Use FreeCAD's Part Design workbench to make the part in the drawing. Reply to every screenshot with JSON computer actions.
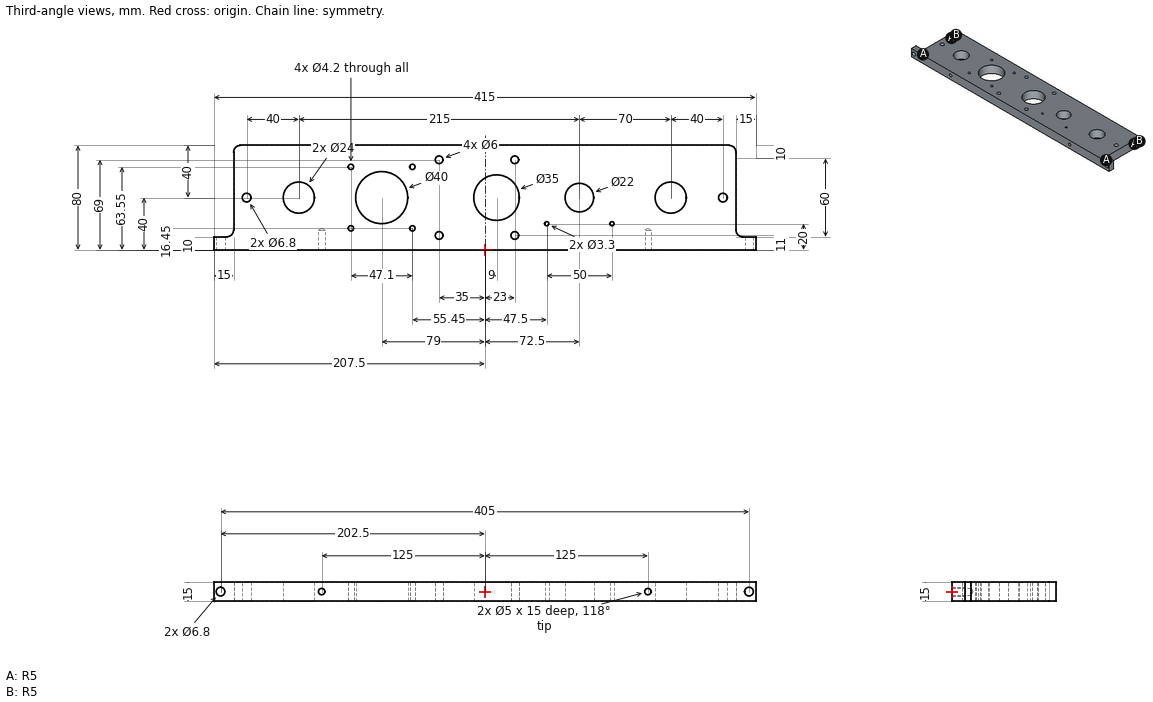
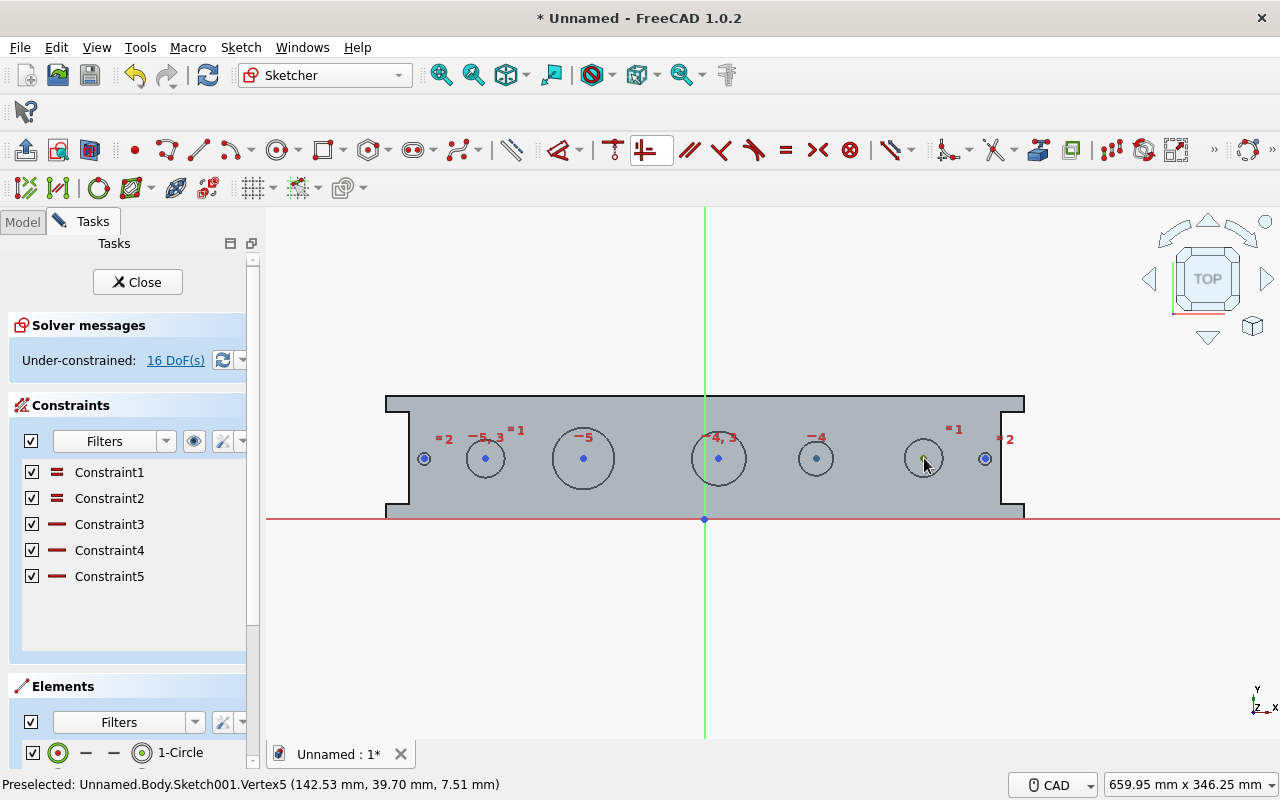
{"action": "left_click", "coordinate": [668, 150]}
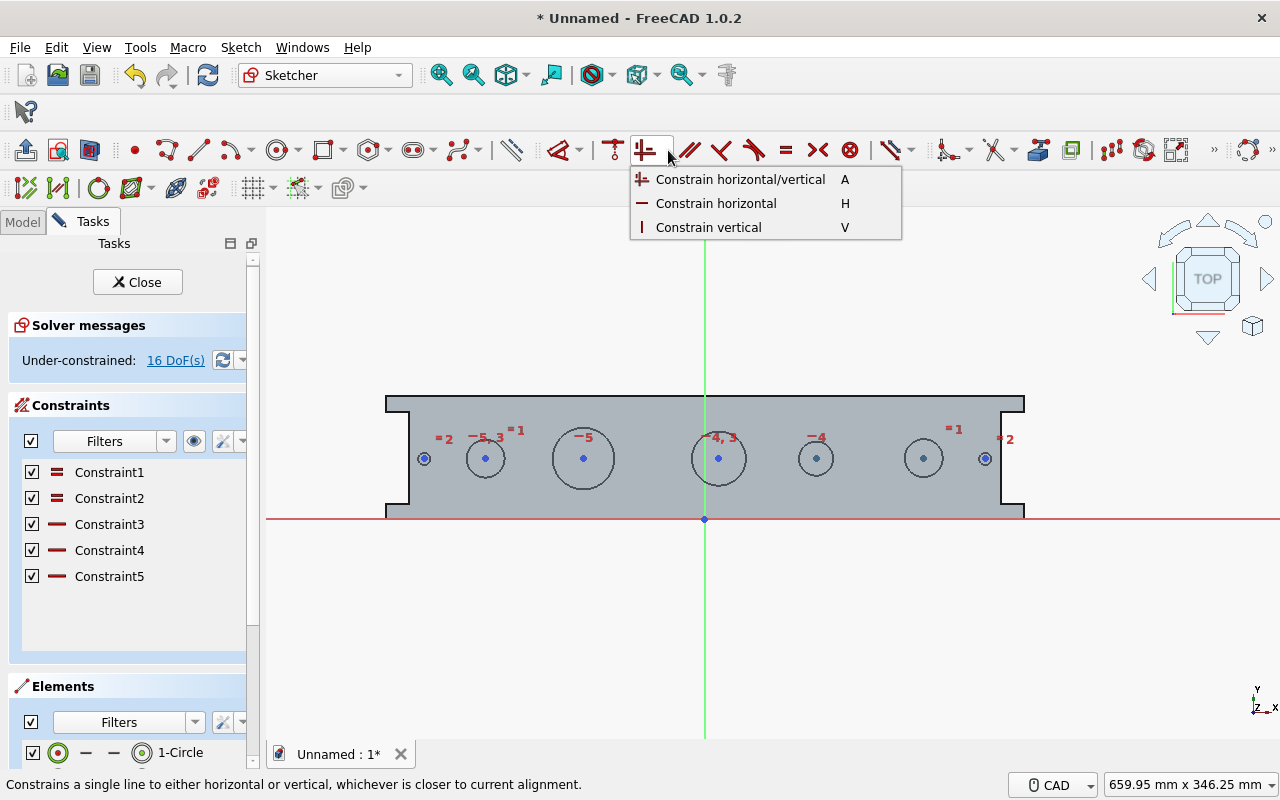
{"action": "left_click", "coordinate": [766, 203]}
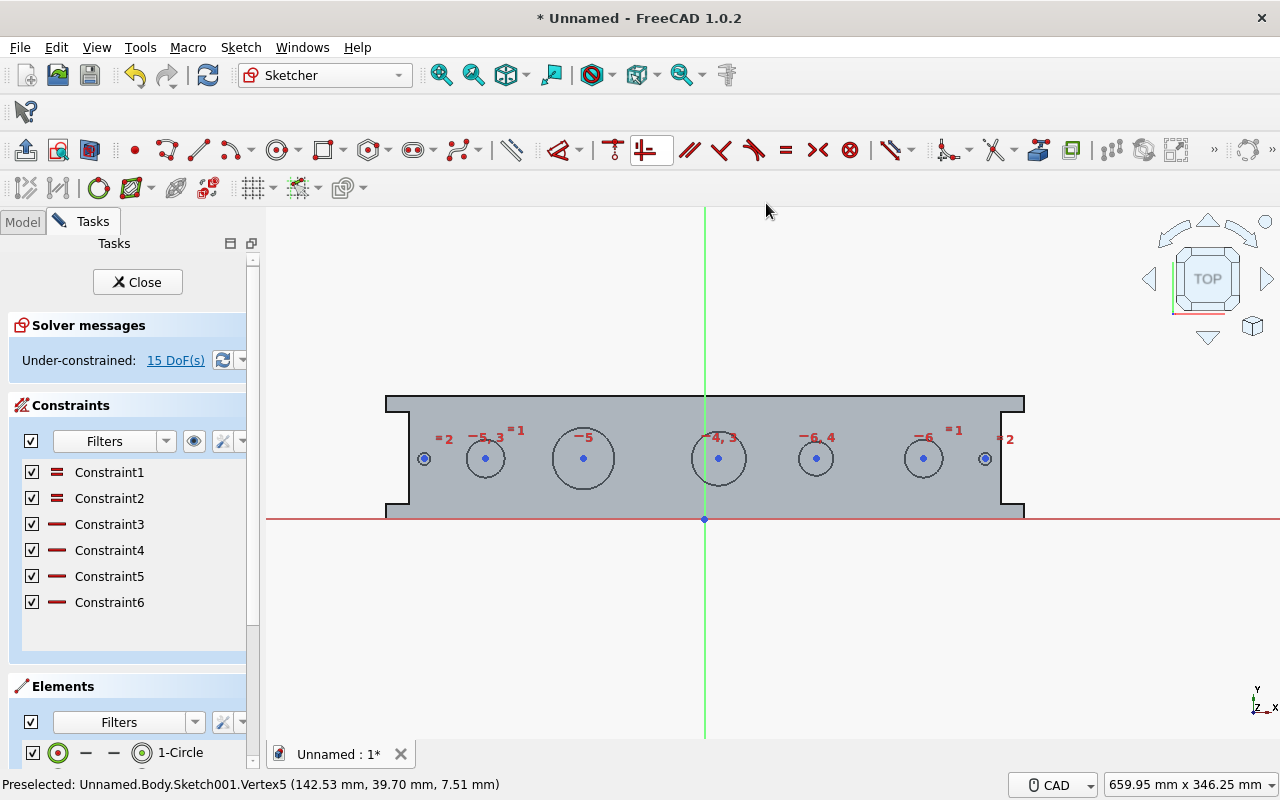
{"action": "left_click", "coordinate": [486, 459]}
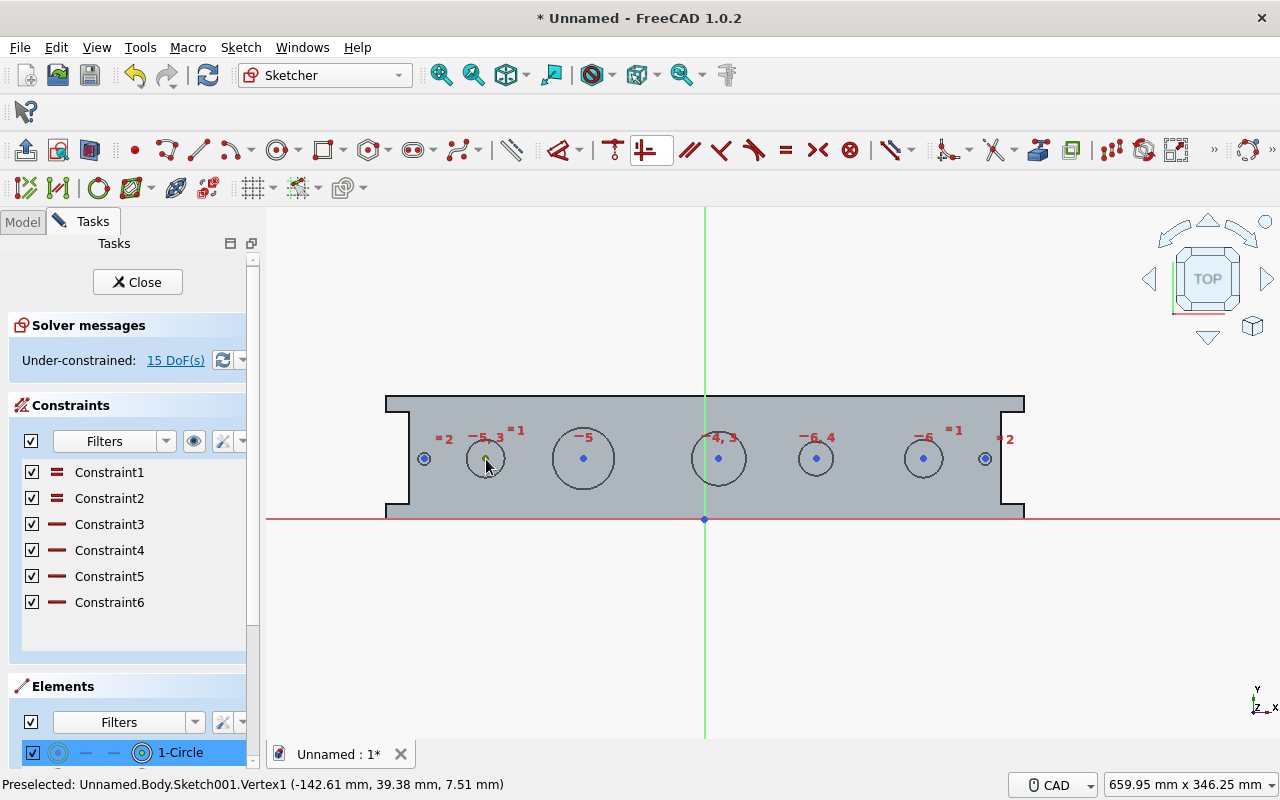
{"action": "left_click", "coordinate": [424, 459]}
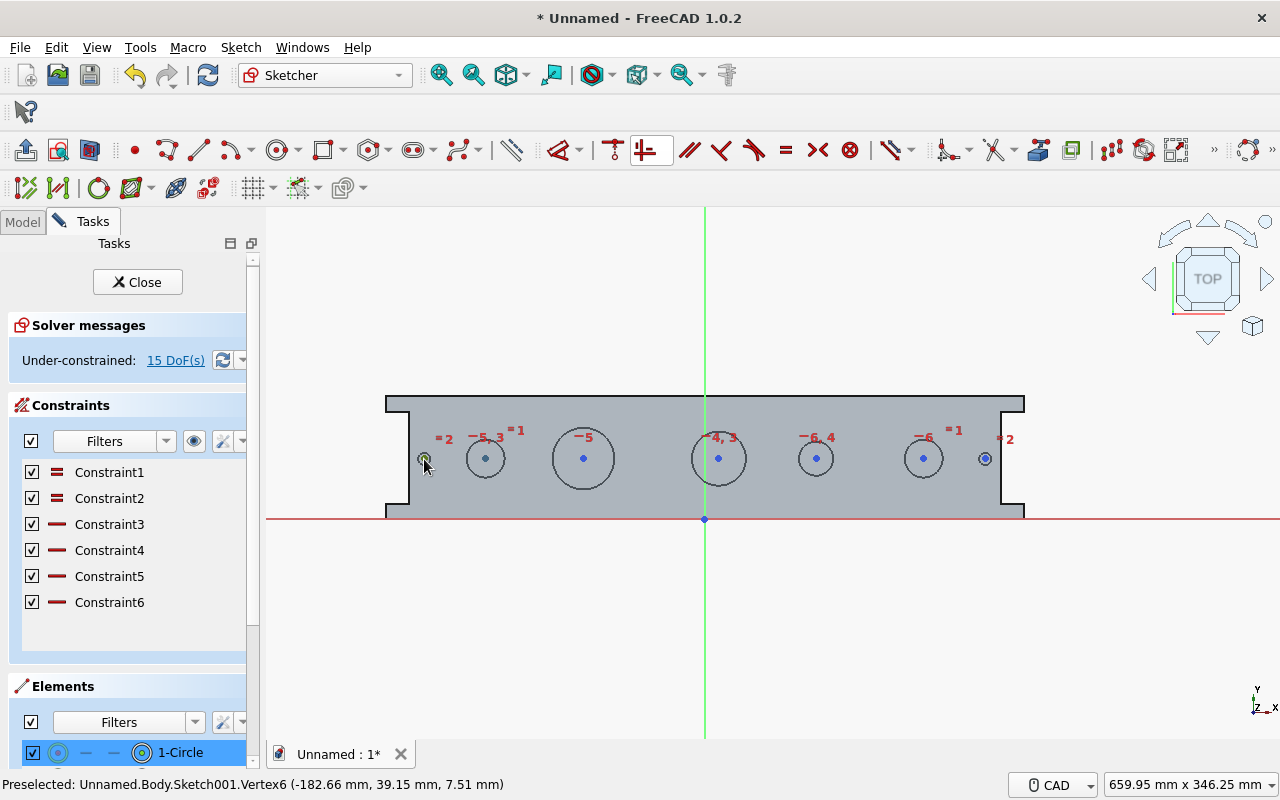
{"action": "left_click", "coordinate": [668, 150]}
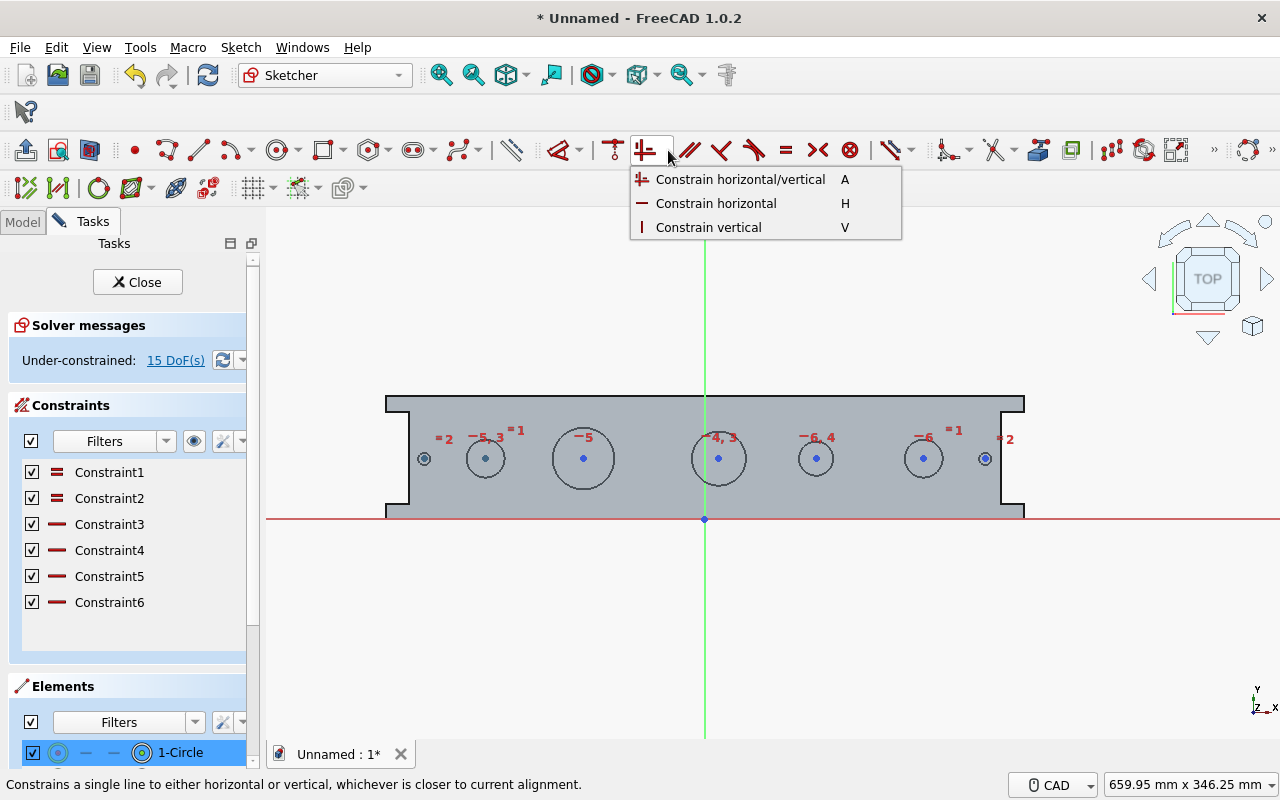
{"action": "left_click", "coordinate": [766, 203]}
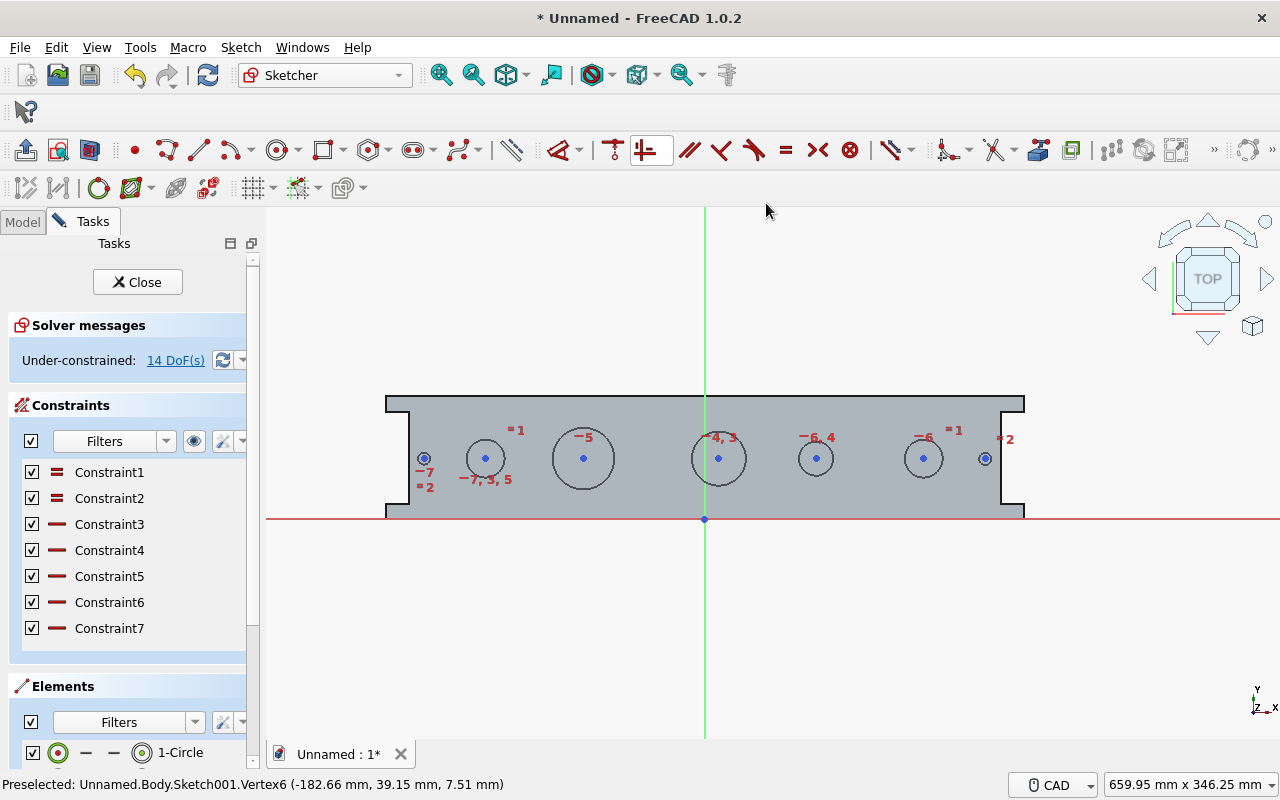
{"action": "left_click", "coordinate": [924, 459]}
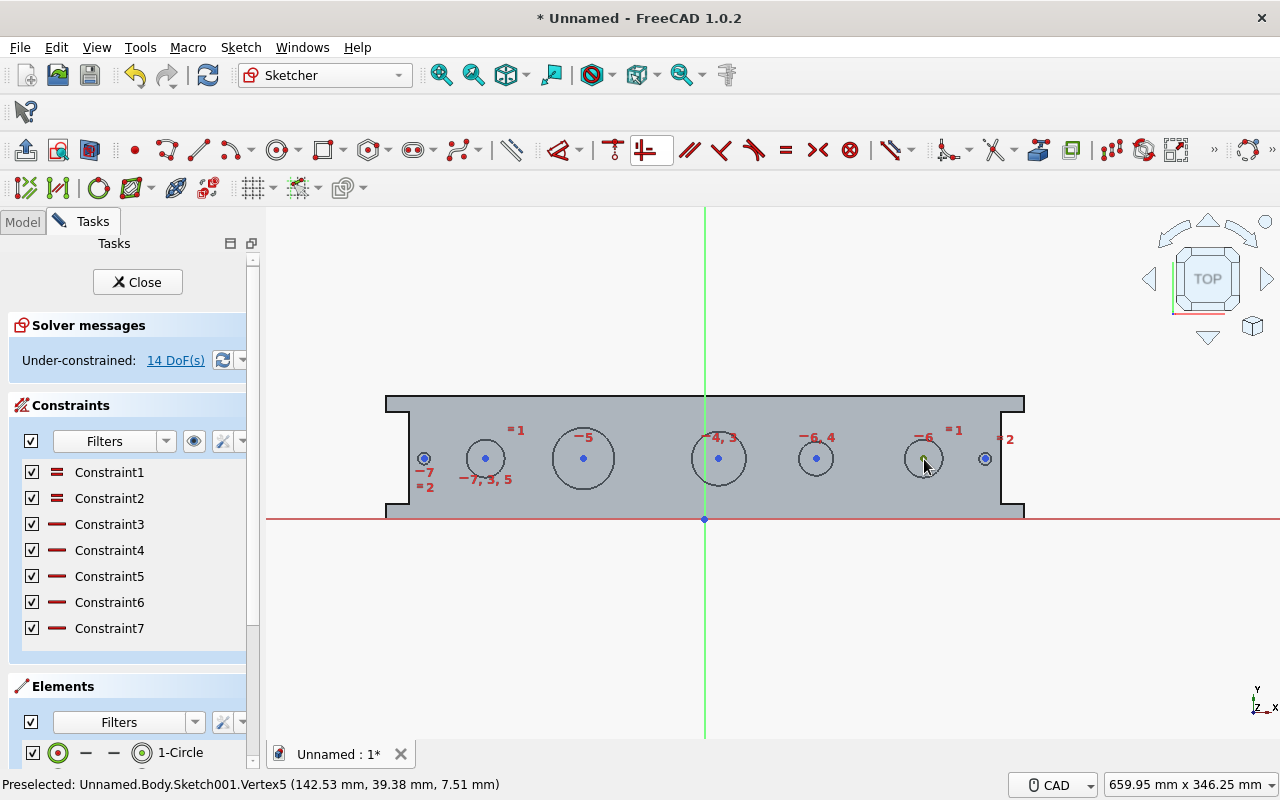
{"action": "left_click", "coordinate": [985, 459]}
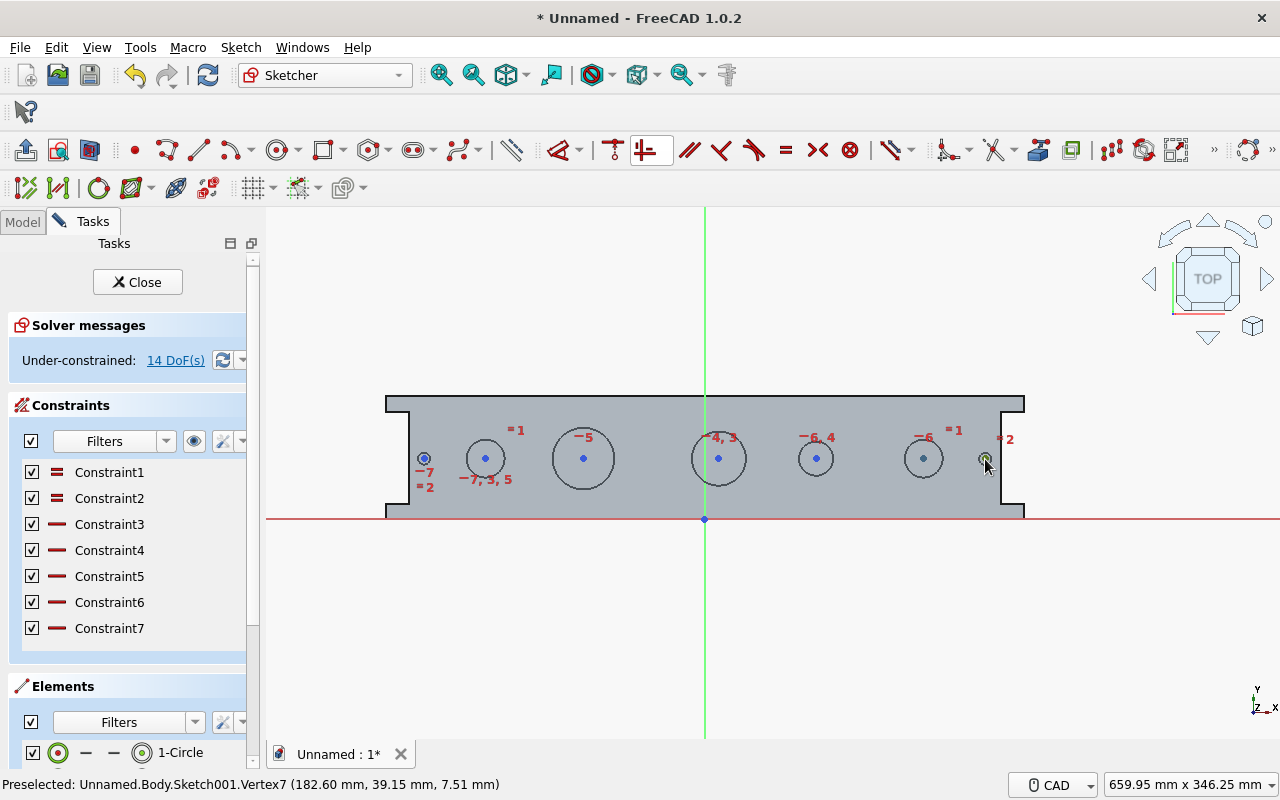
{"action": "left_click", "coordinate": [668, 150]}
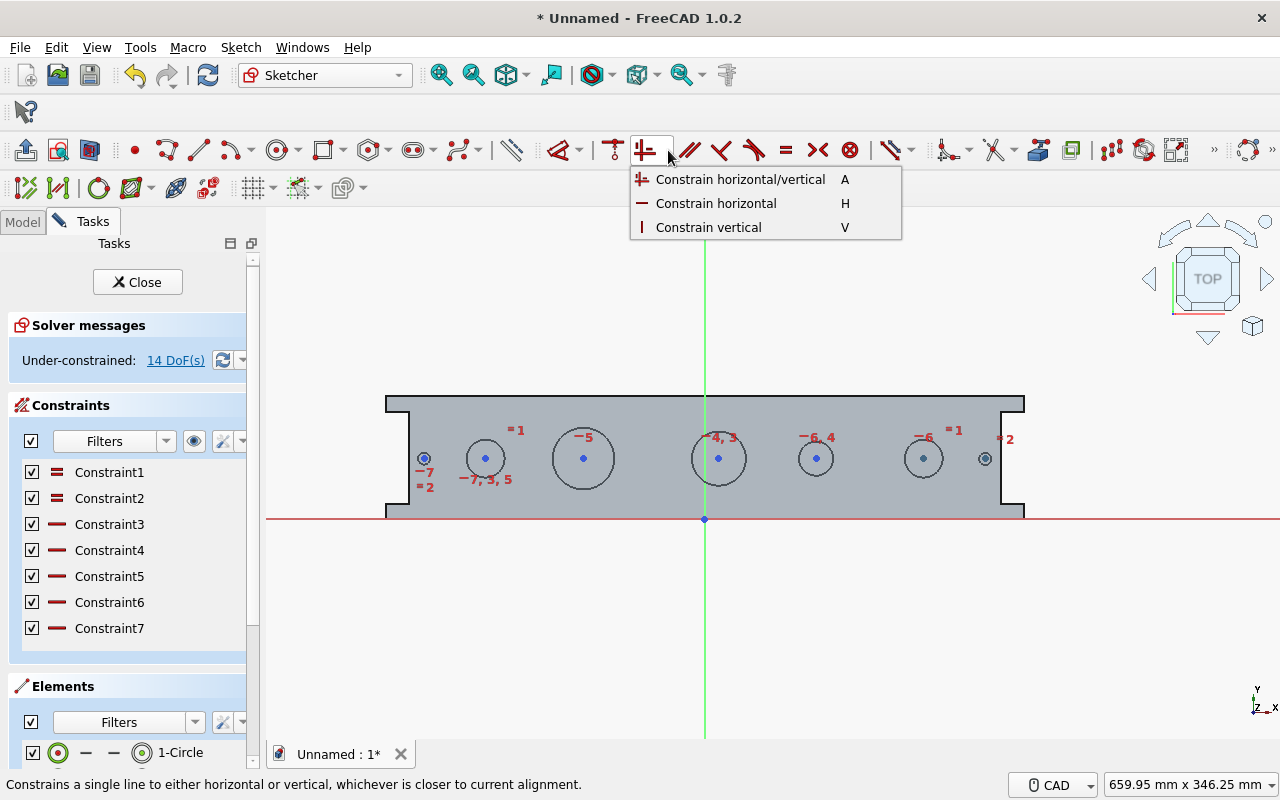
{"action": "left_click", "coordinate": [766, 203]}